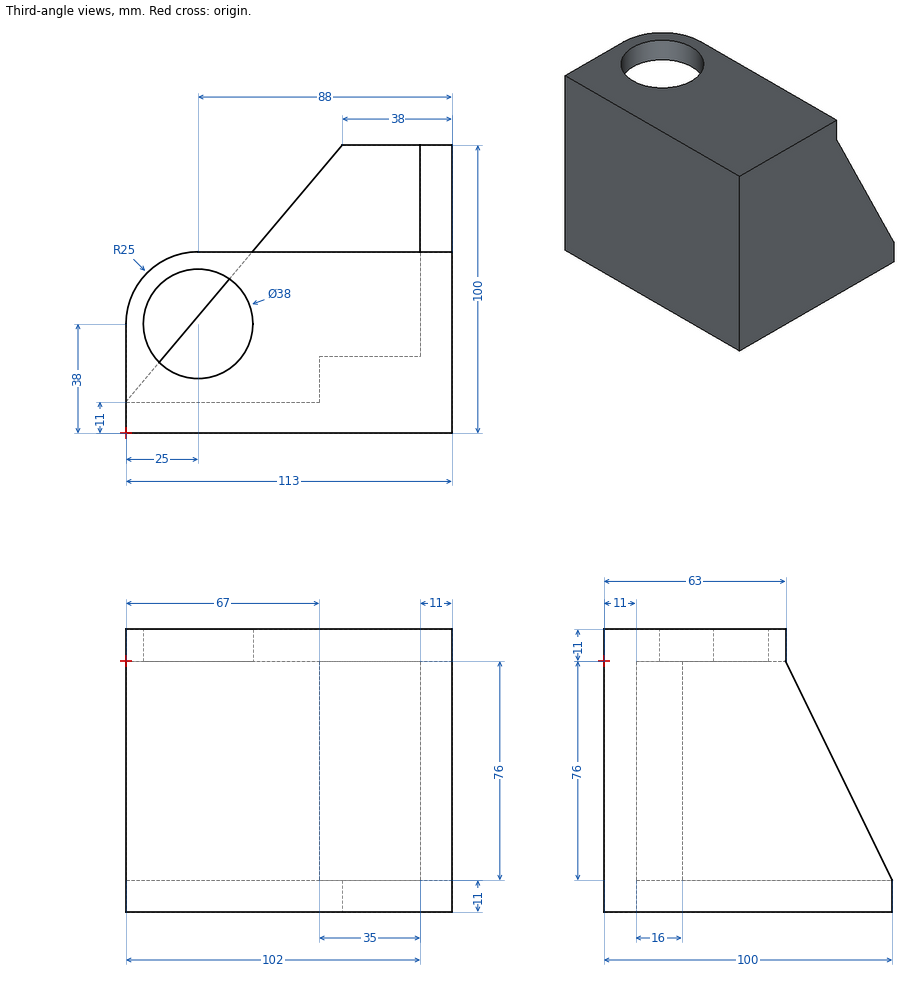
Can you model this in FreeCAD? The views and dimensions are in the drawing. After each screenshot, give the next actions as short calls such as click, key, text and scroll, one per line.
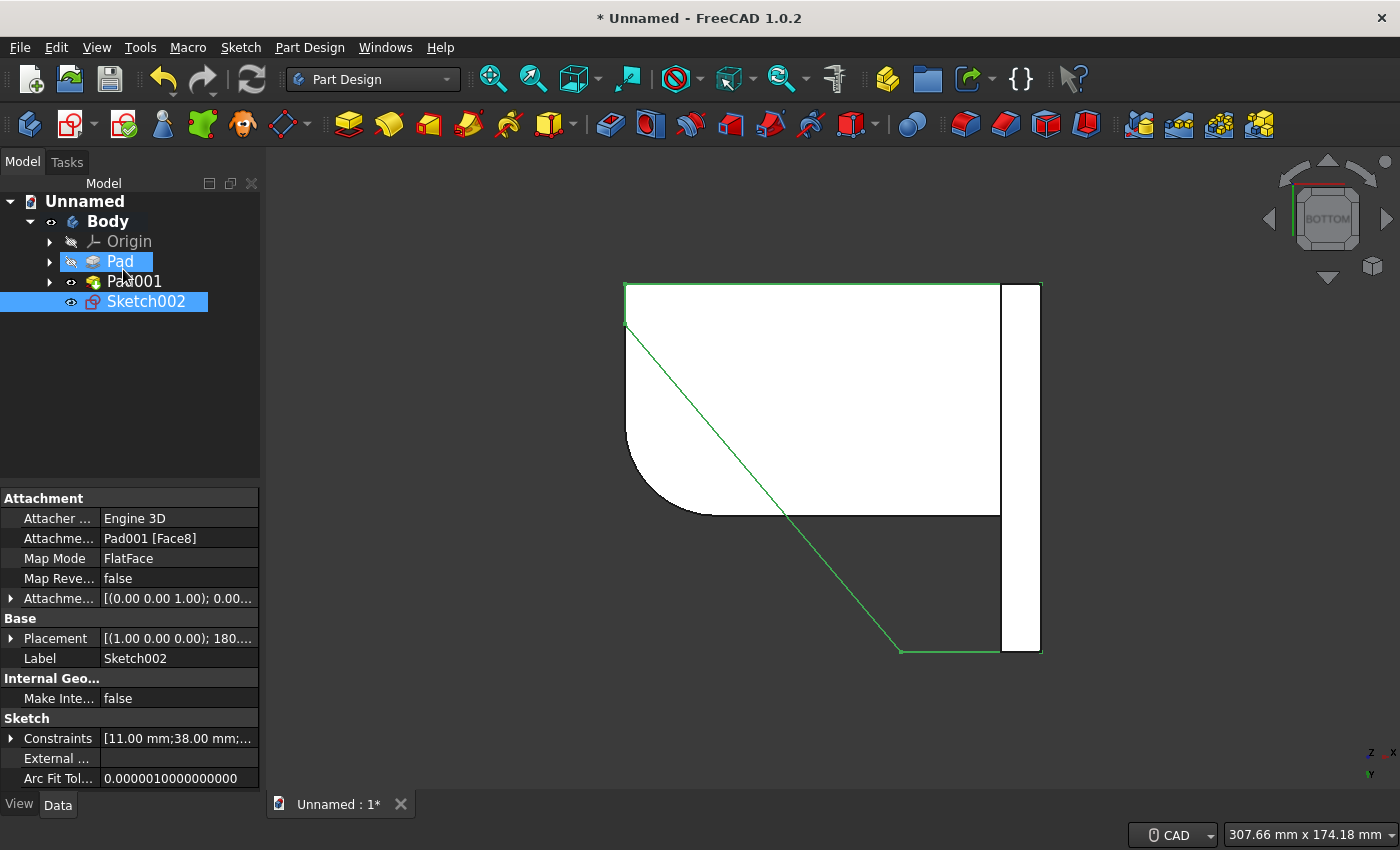
click(350, 124)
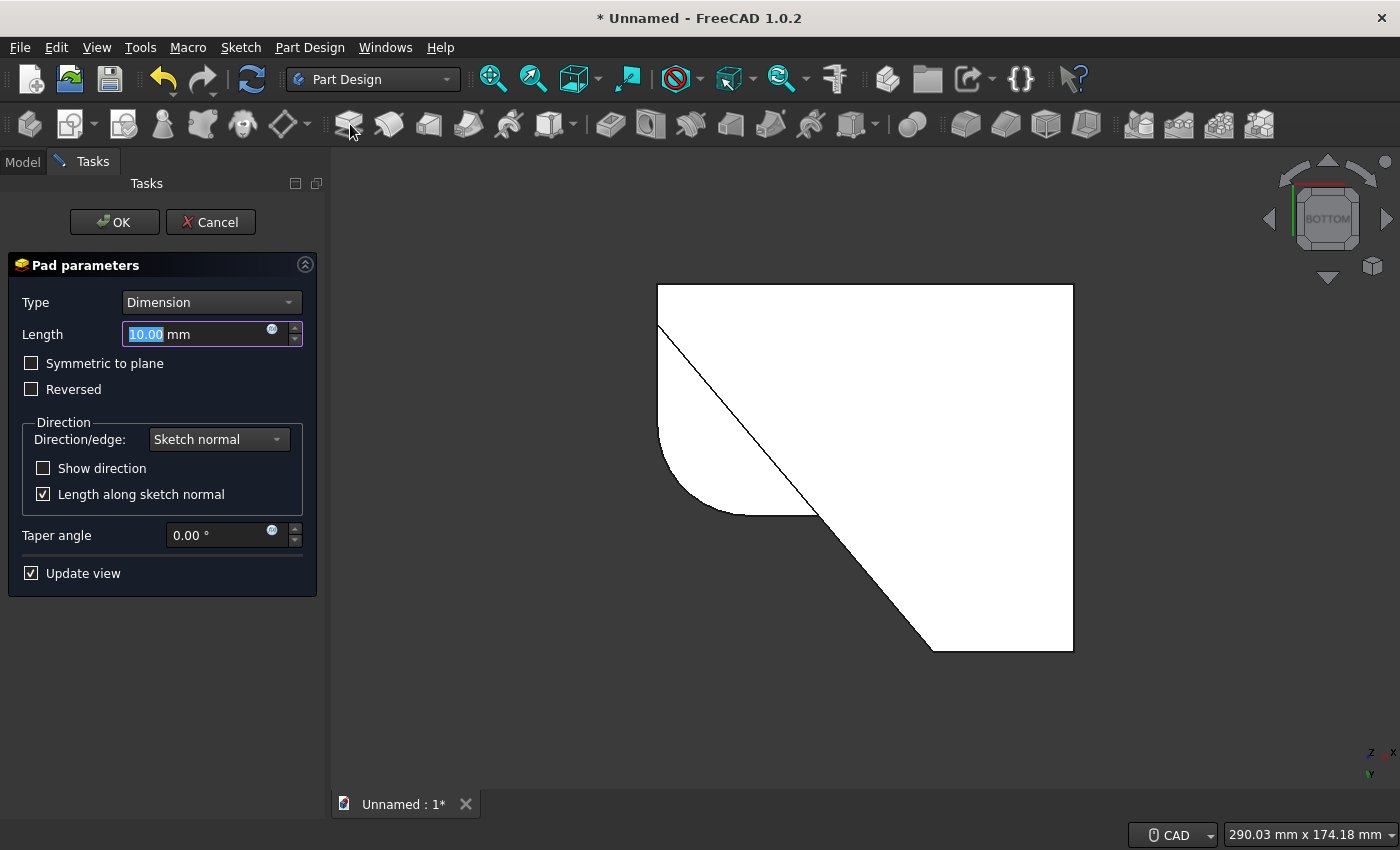
text(11)
key(Tab)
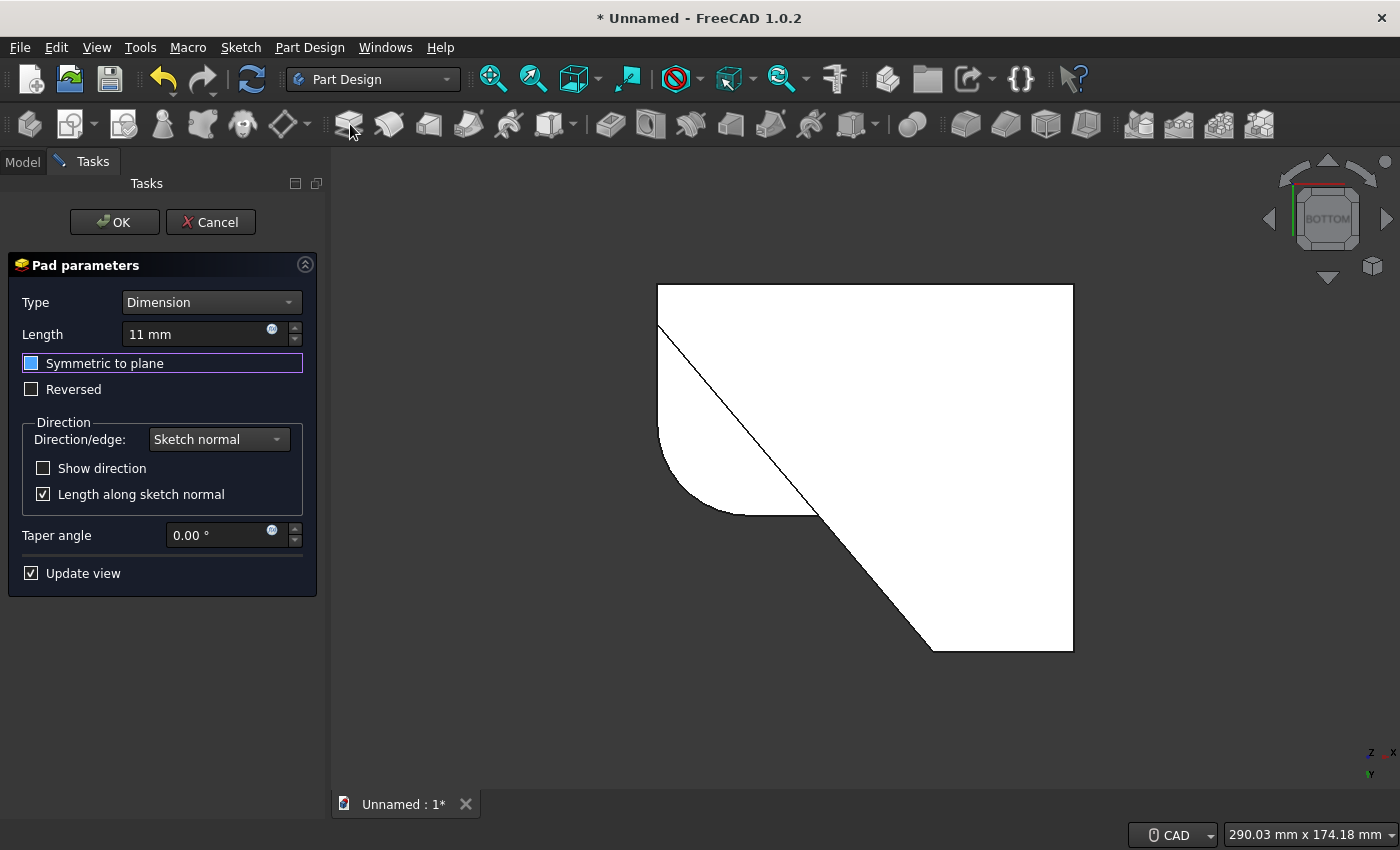
click(115, 222)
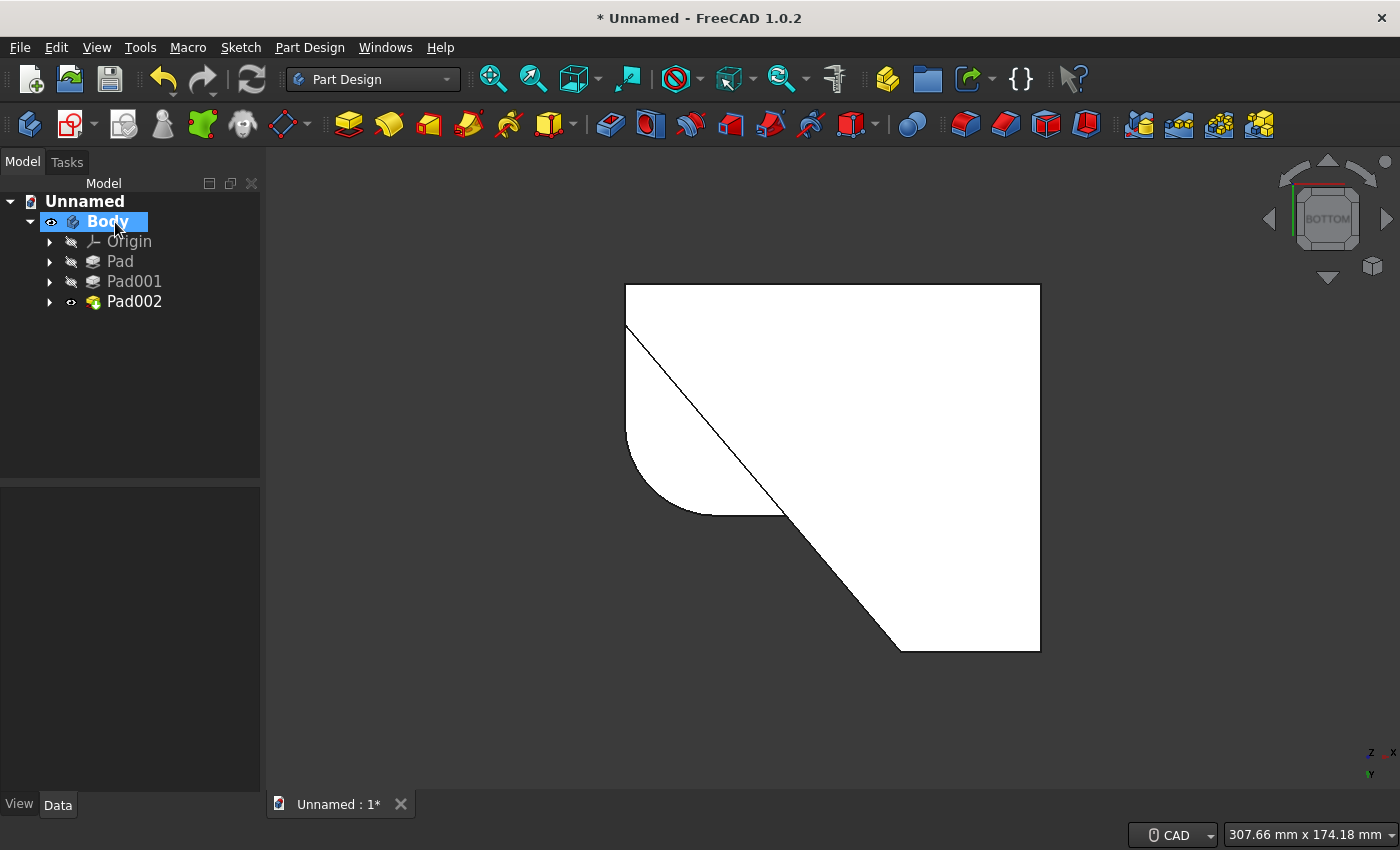
click(70, 124)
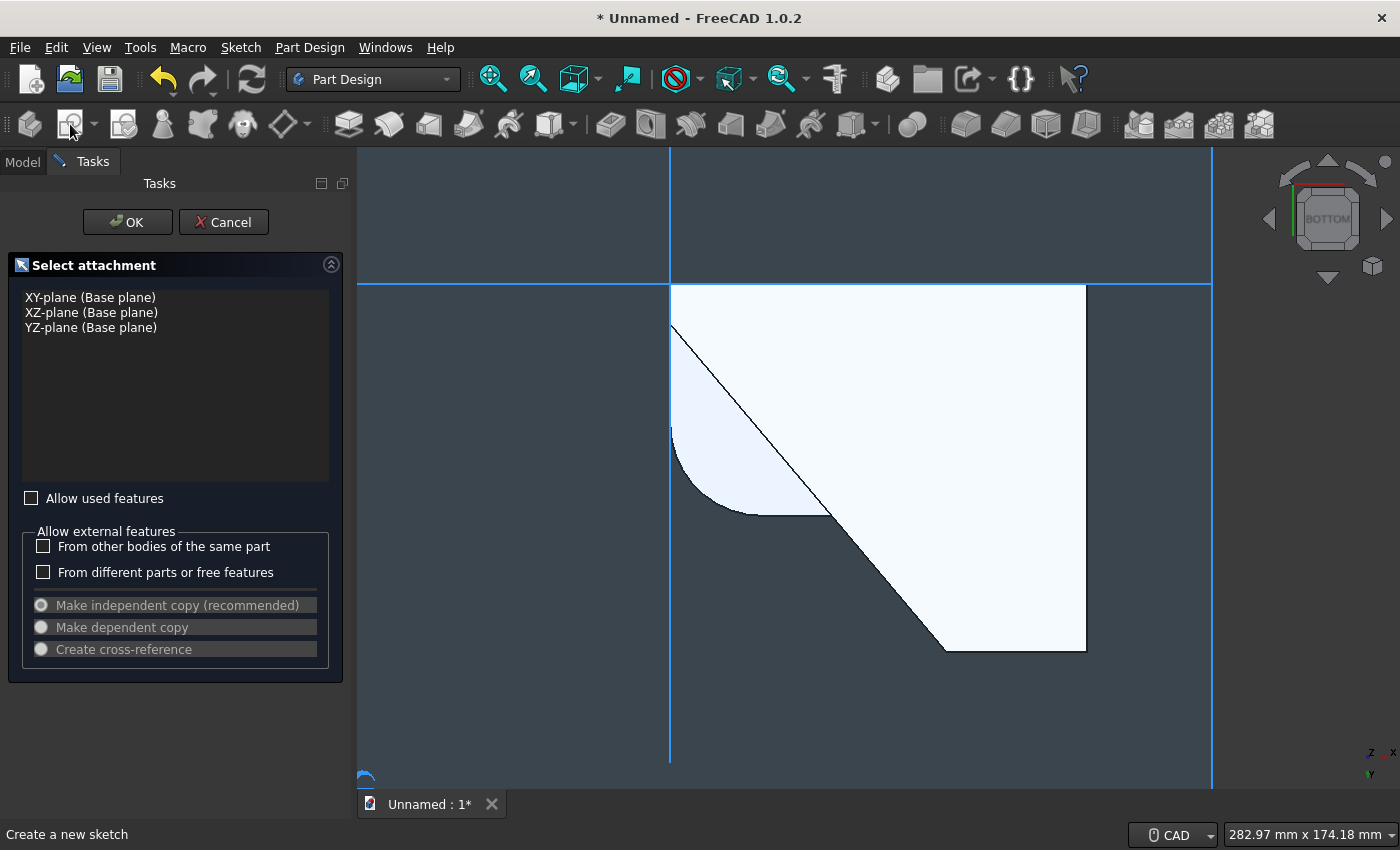
click(82, 312)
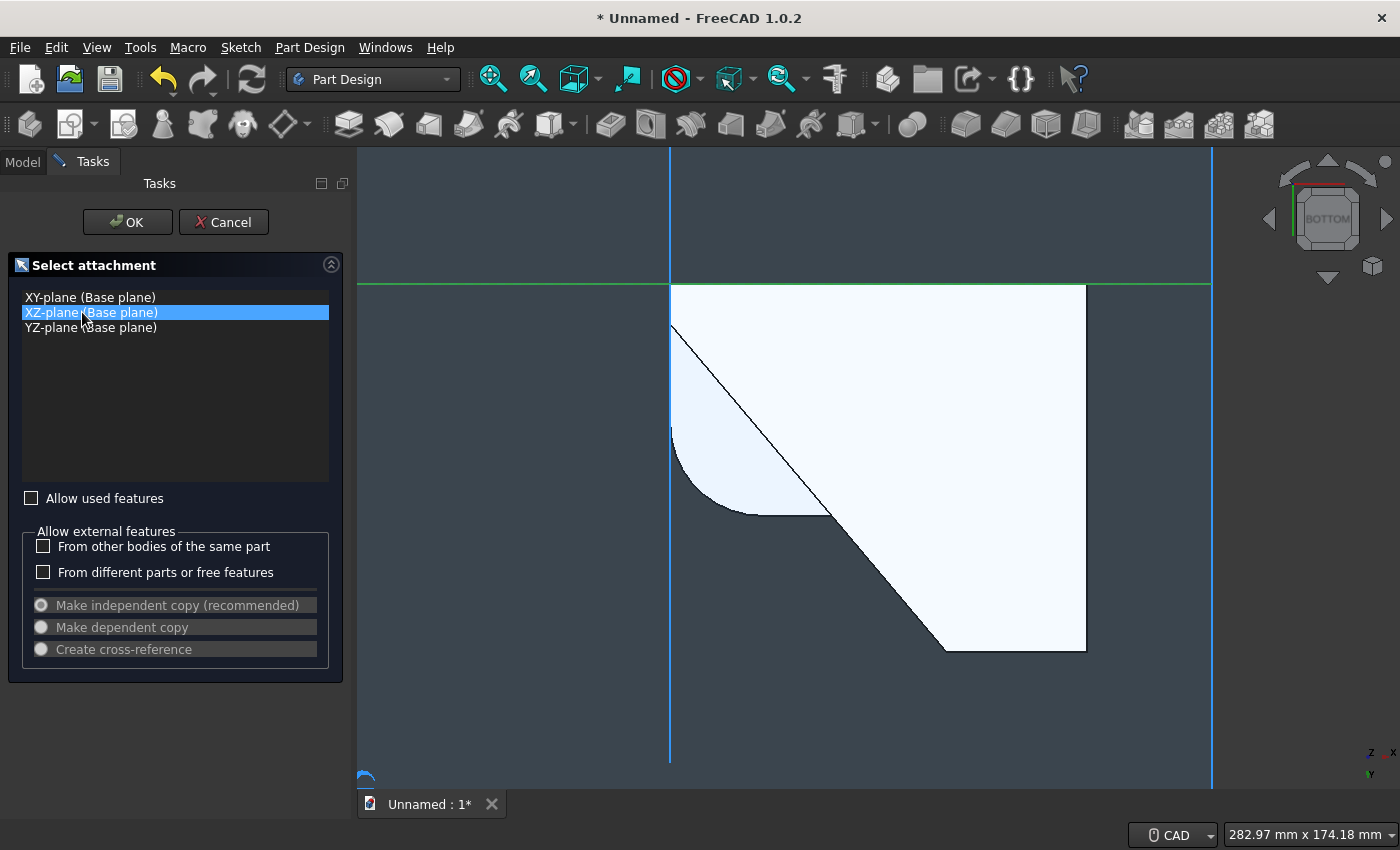
click(128, 222)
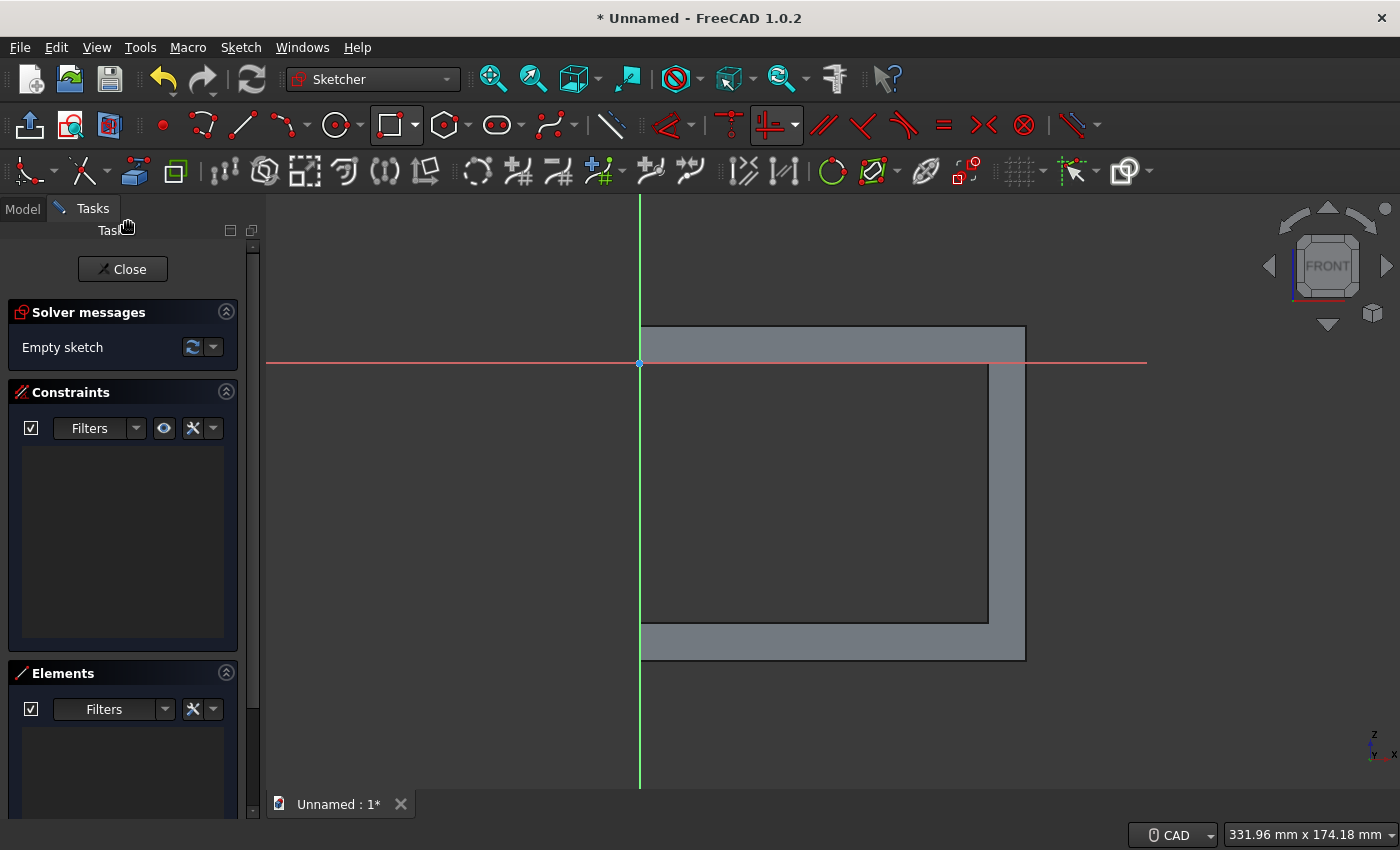
scroll(915, 497, up, 2)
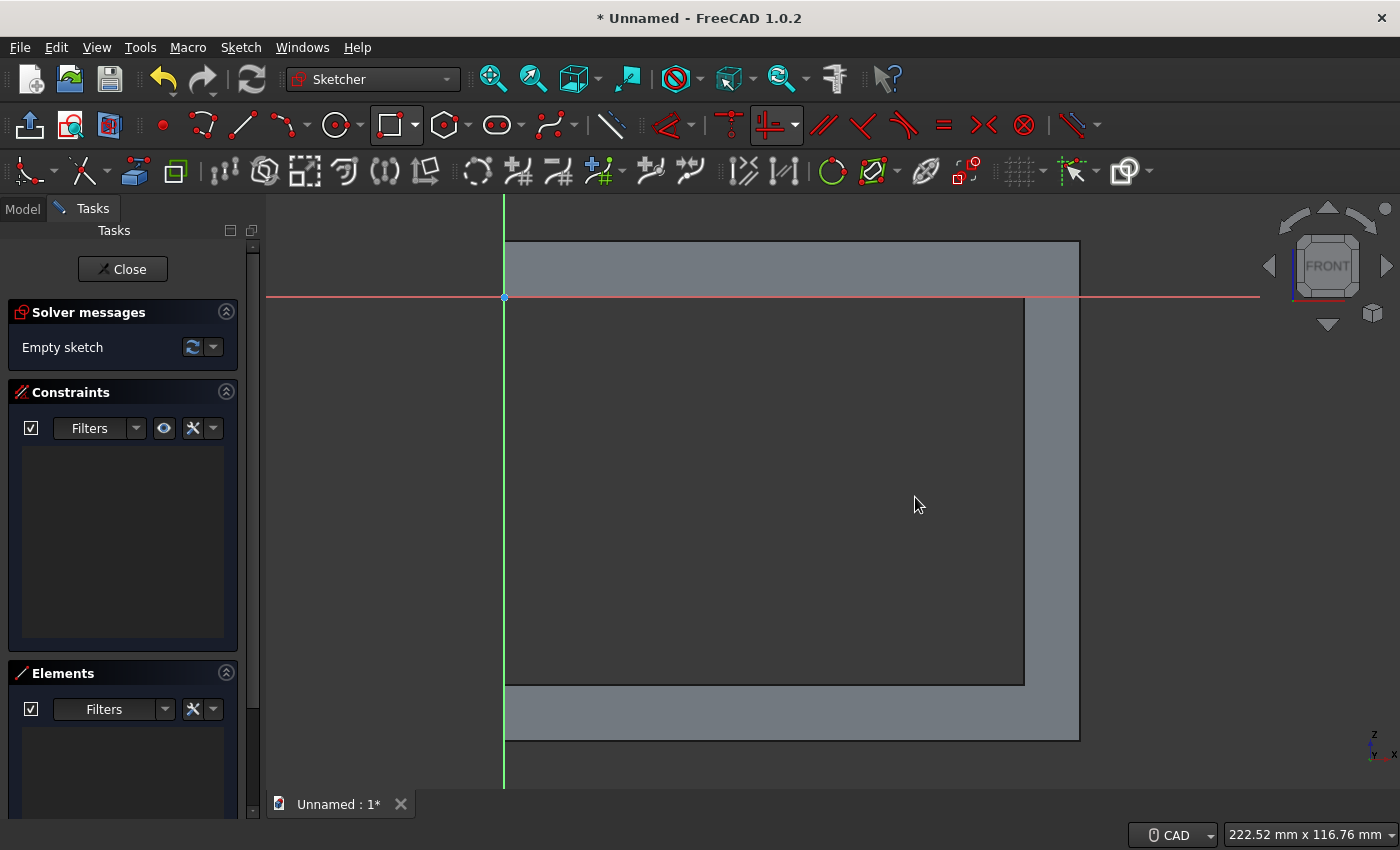
key(g)
key(r)